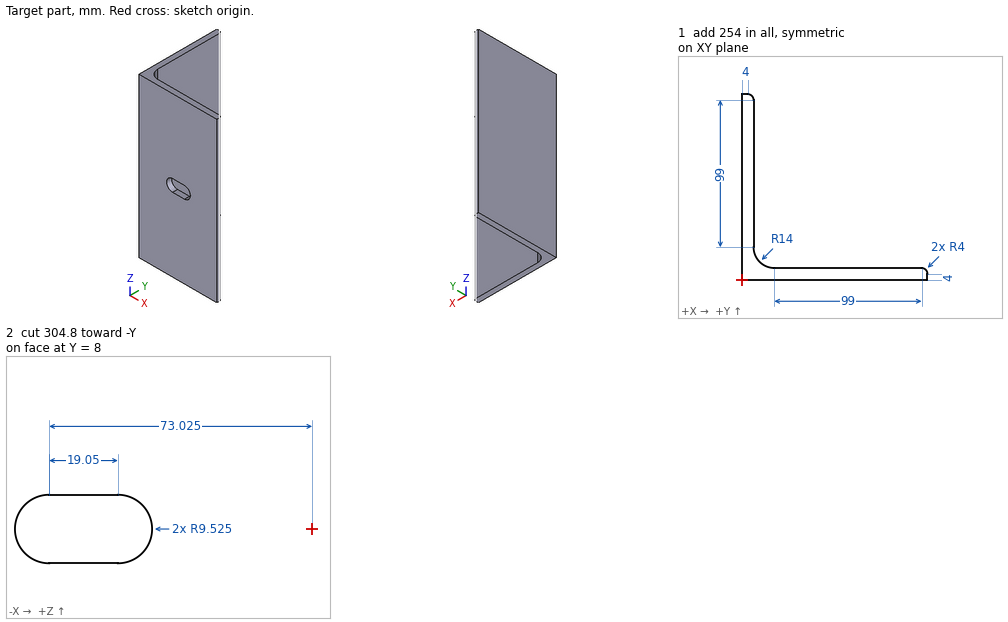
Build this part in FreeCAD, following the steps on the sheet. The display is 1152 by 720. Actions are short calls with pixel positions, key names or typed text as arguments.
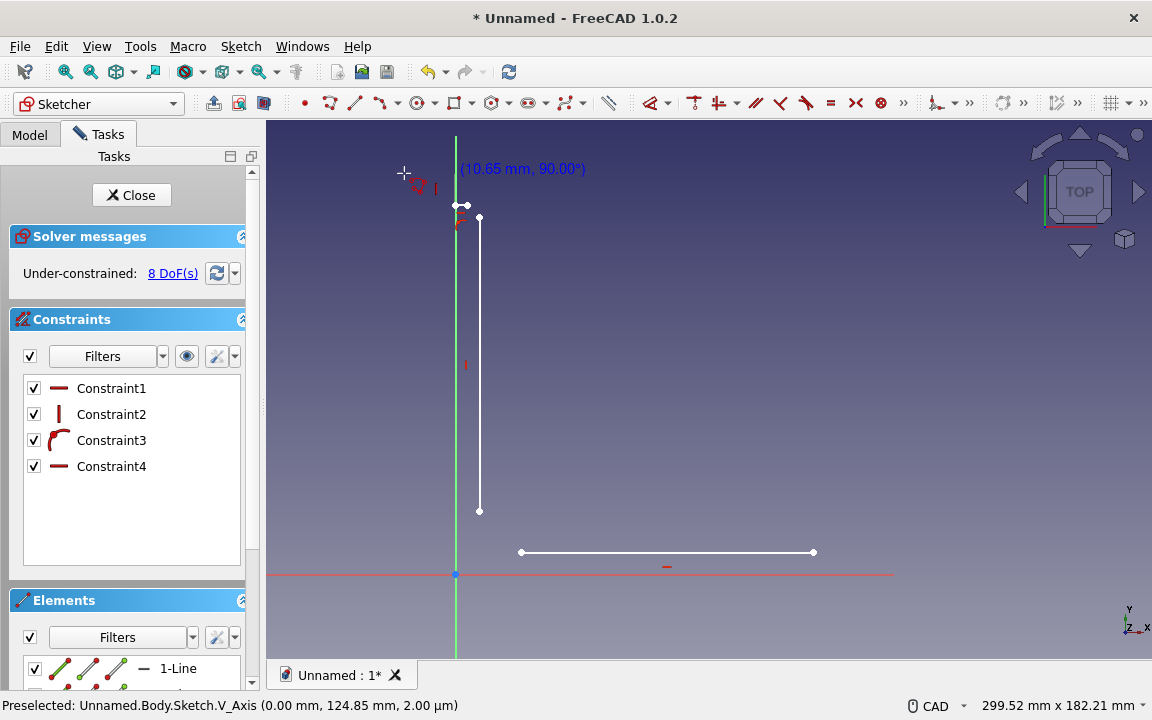
click(456, 575)
click(826, 566)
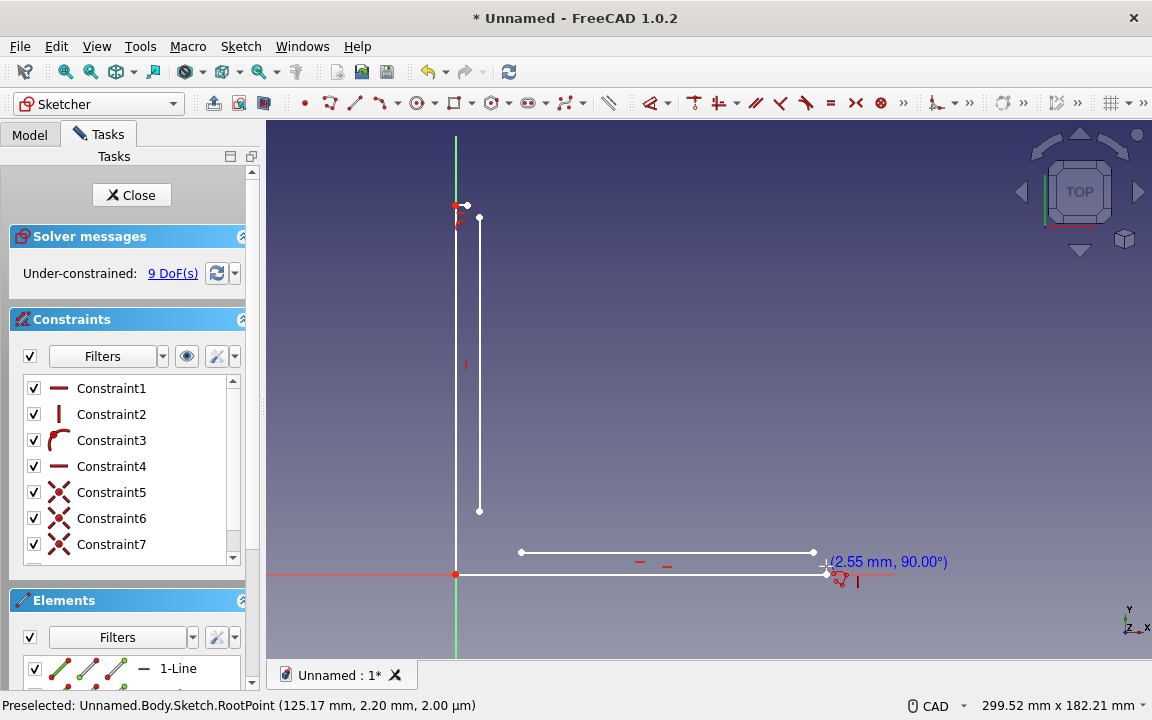
scroll(826, 563, up, 2)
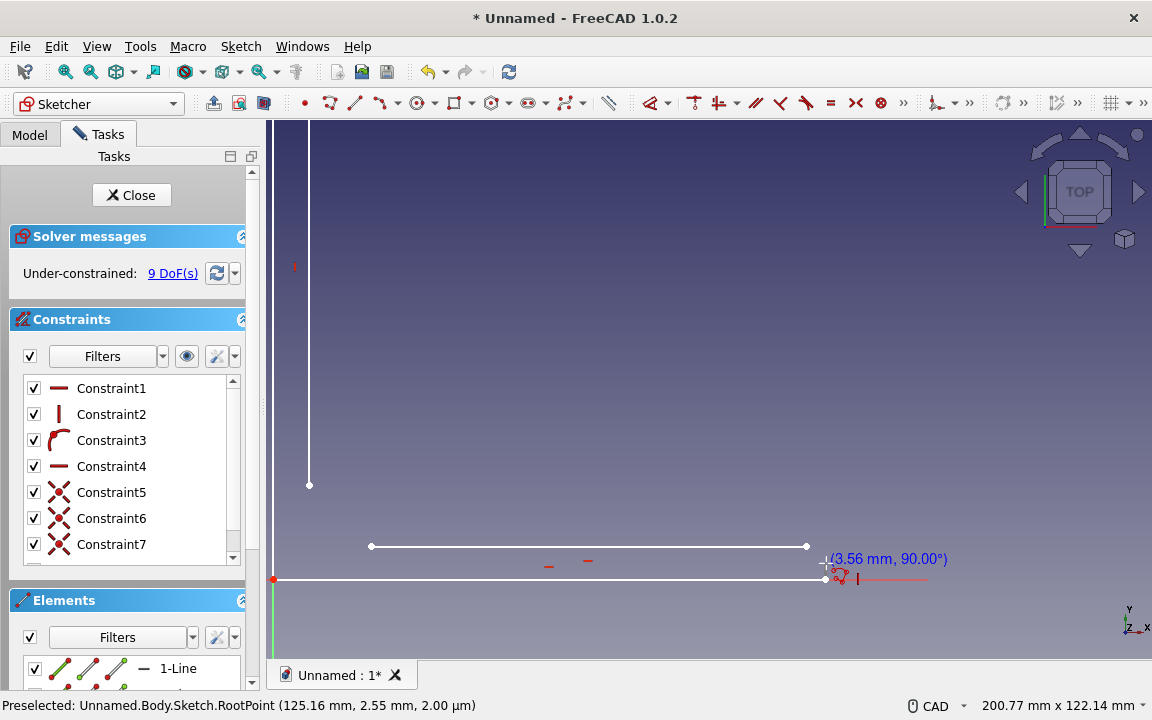
click(826, 562)
right_click(826, 562)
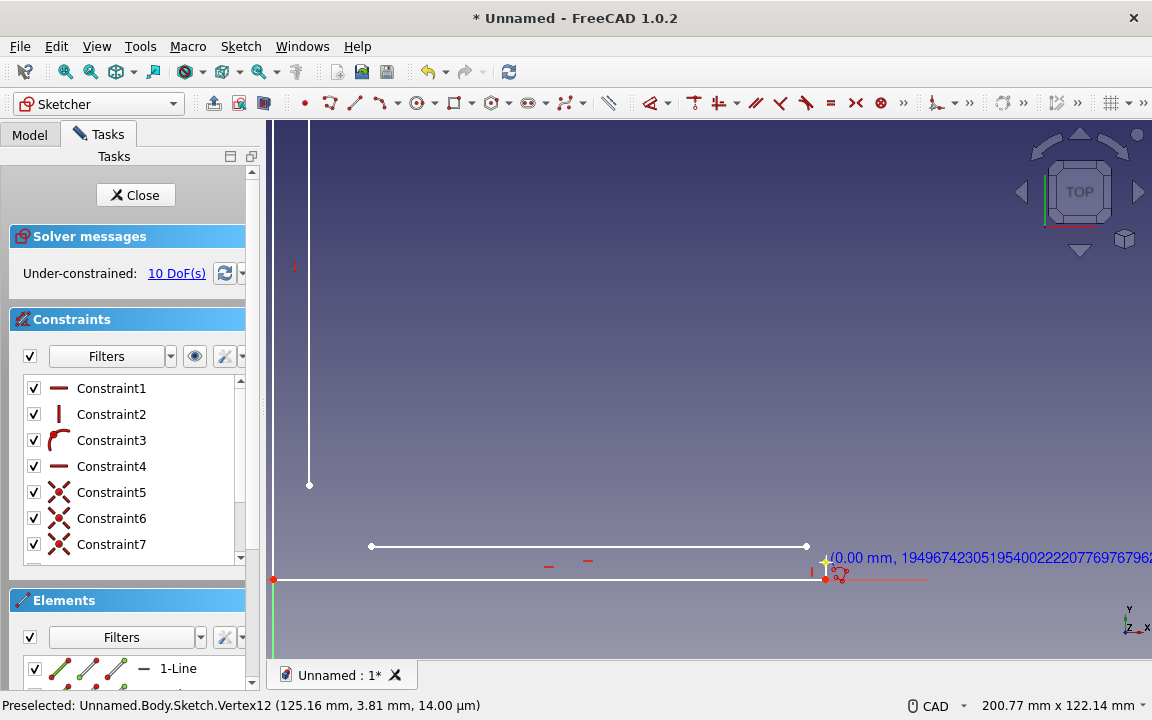
key(g)
key(3)
key(a)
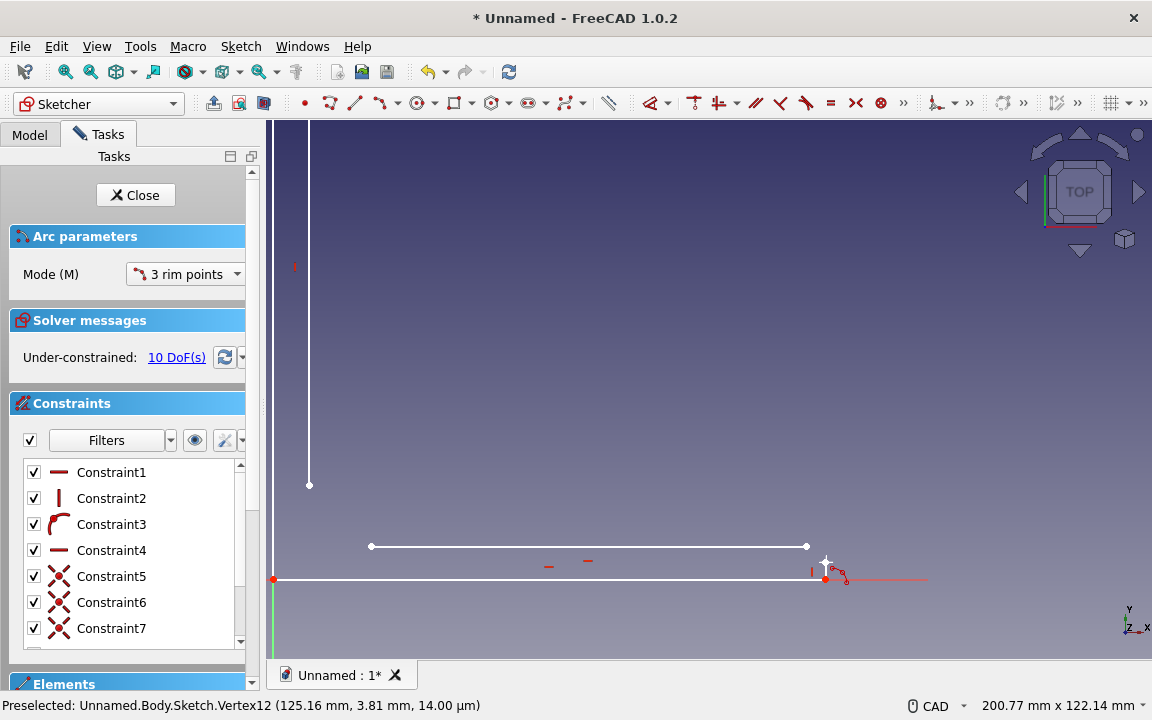
click(371, 547)
click(309, 485)
click(327, 526)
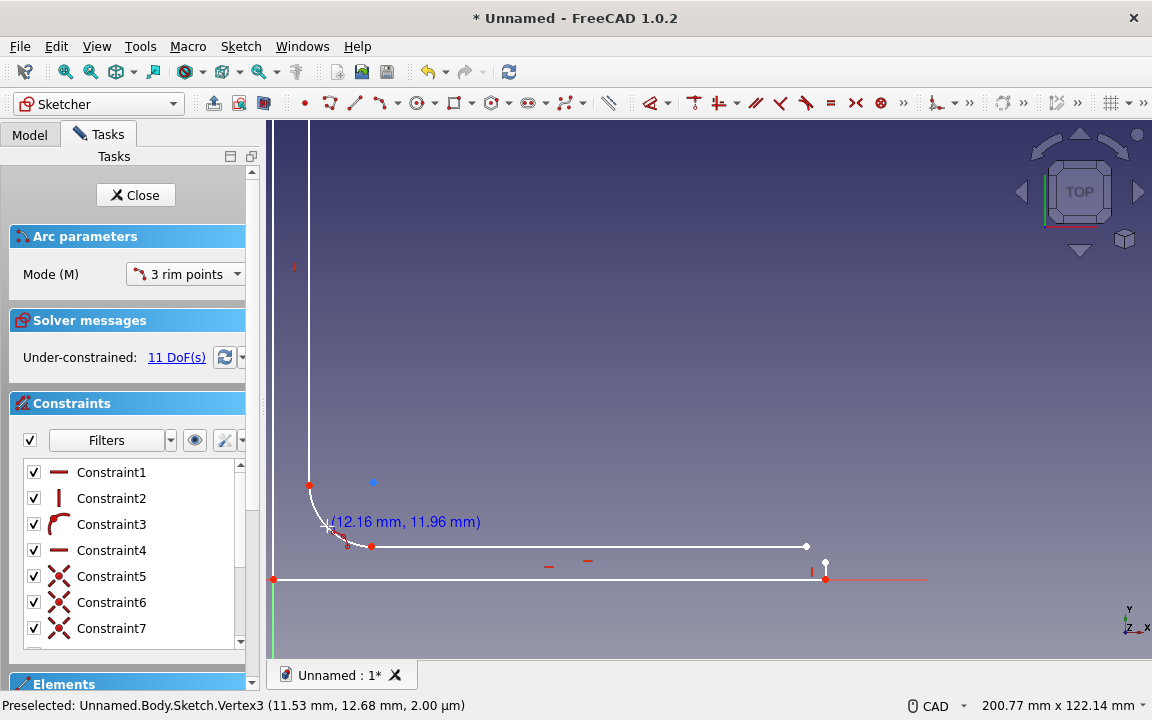
scroll(826, 563, down, 2)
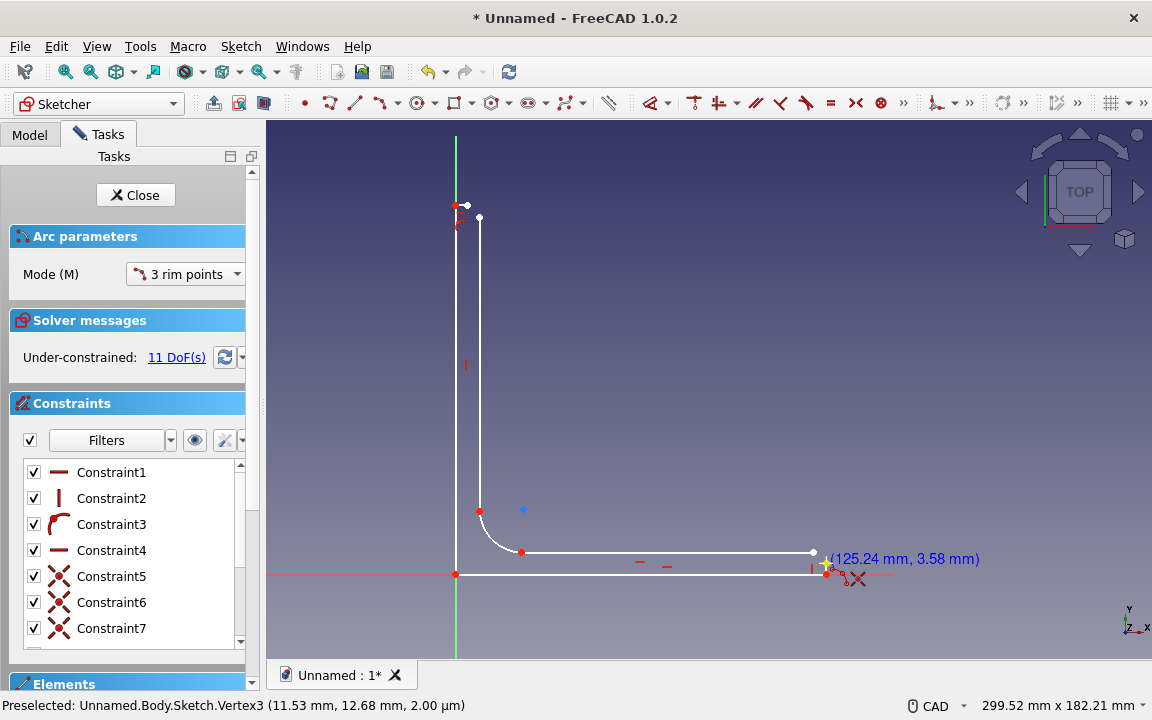
click(480, 218)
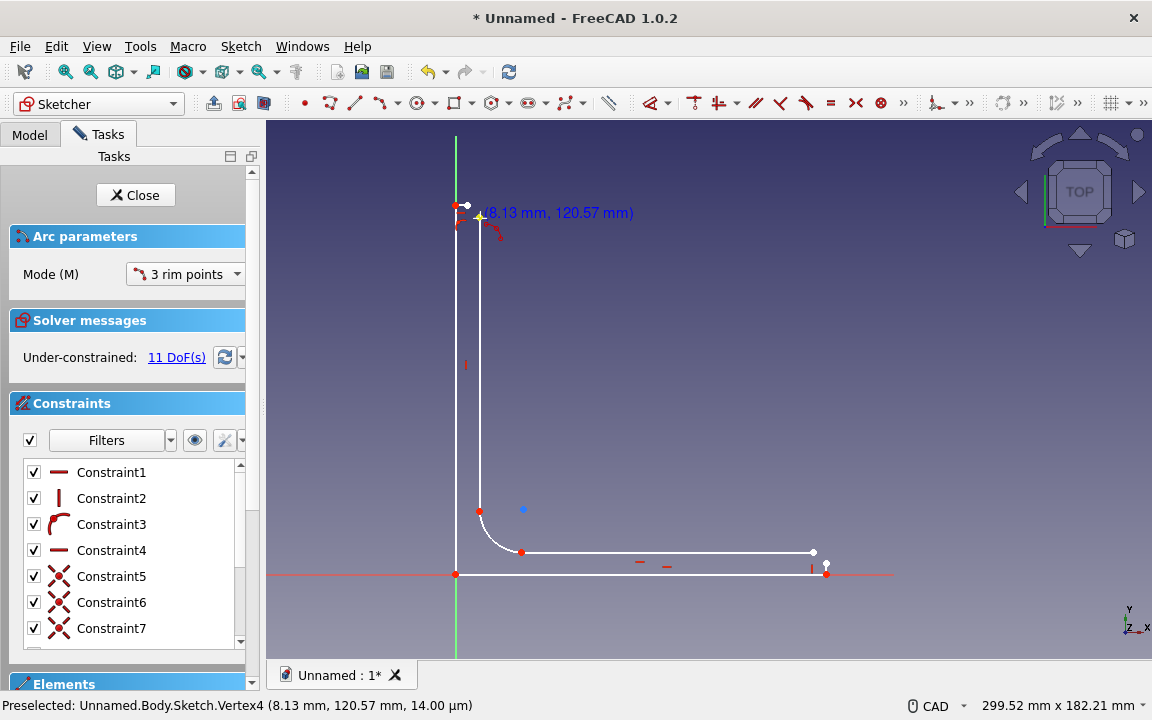
scroll(468, 205, up, 5)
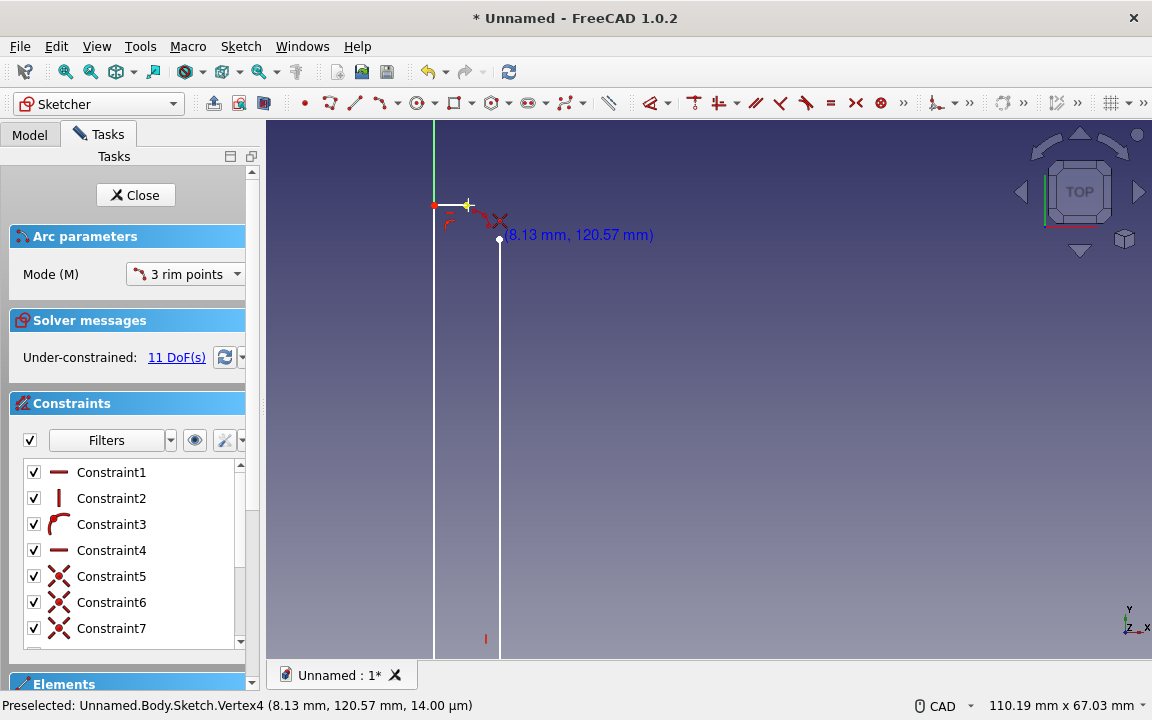
click(467, 205)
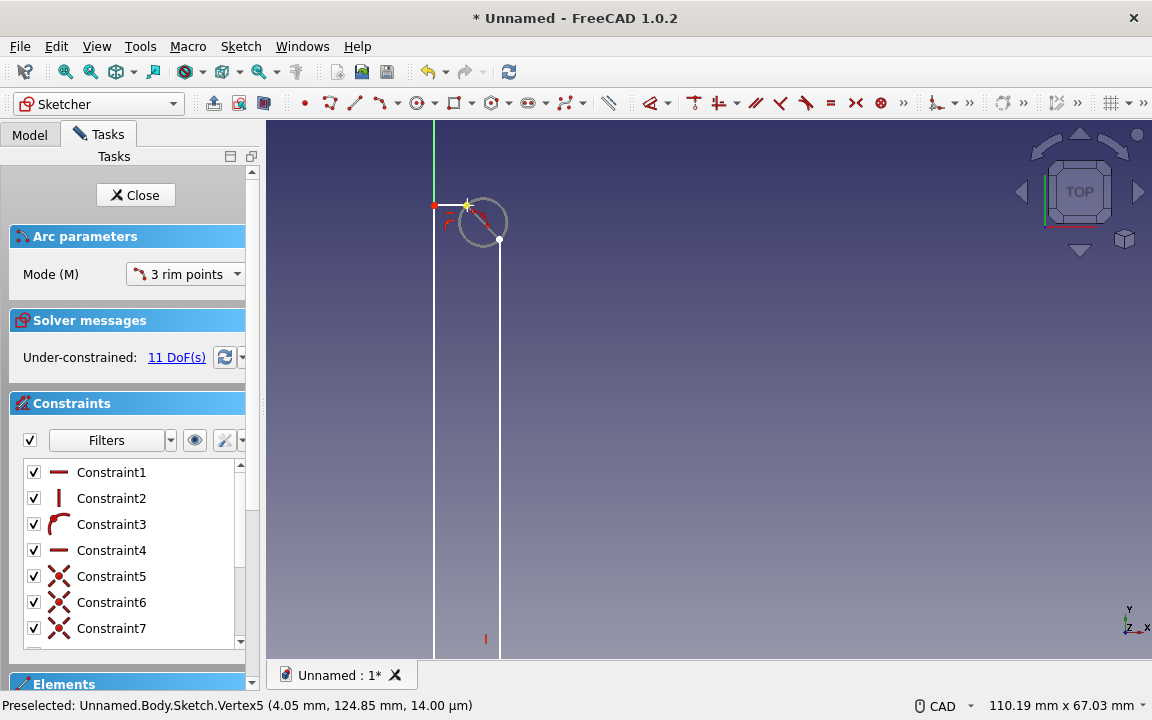
scroll(489, 214, up, 3)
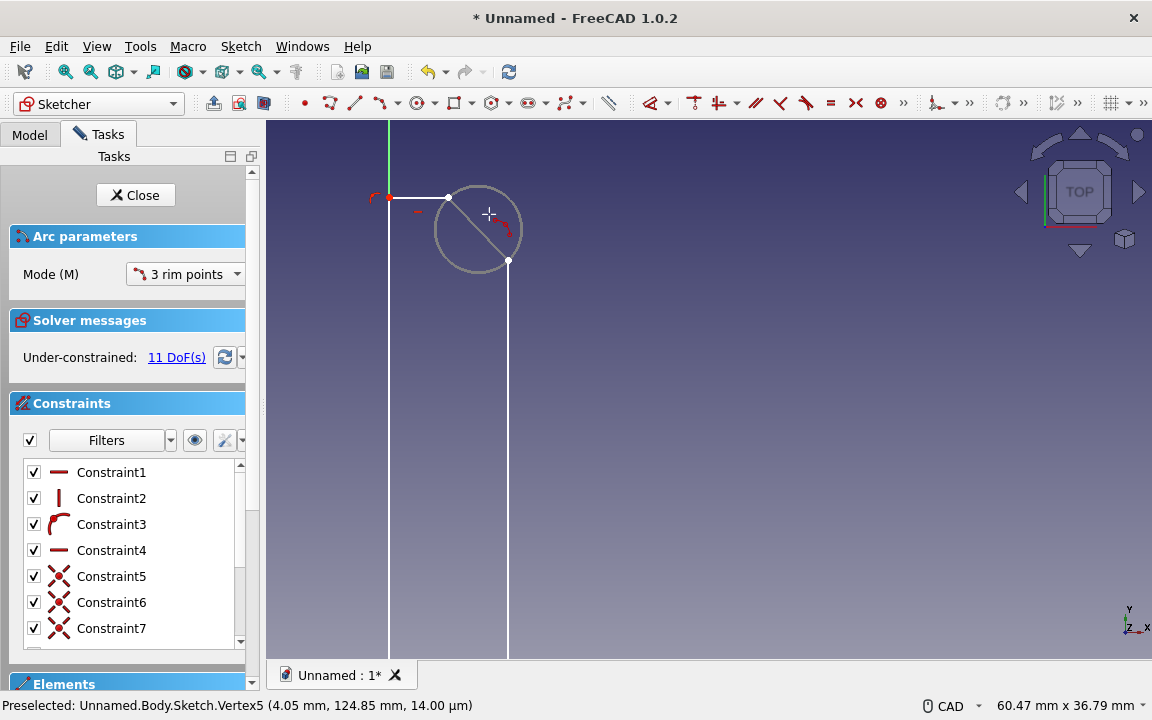
click(489, 213)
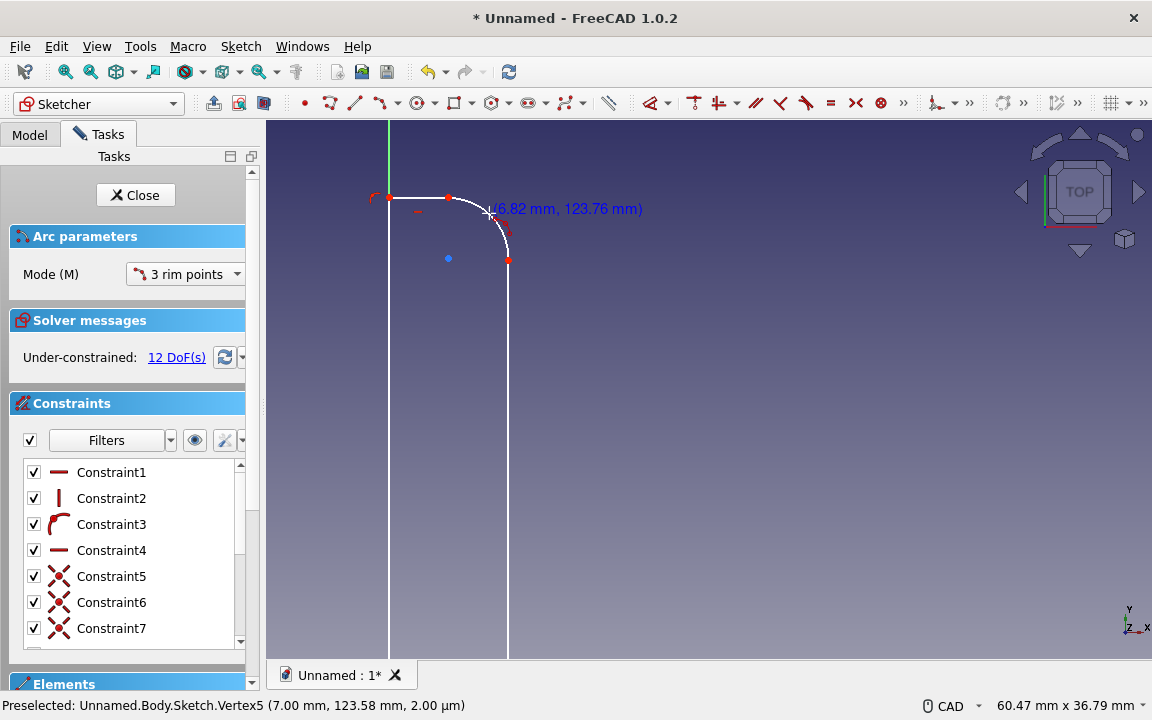
scroll(472, 207, down, 8)